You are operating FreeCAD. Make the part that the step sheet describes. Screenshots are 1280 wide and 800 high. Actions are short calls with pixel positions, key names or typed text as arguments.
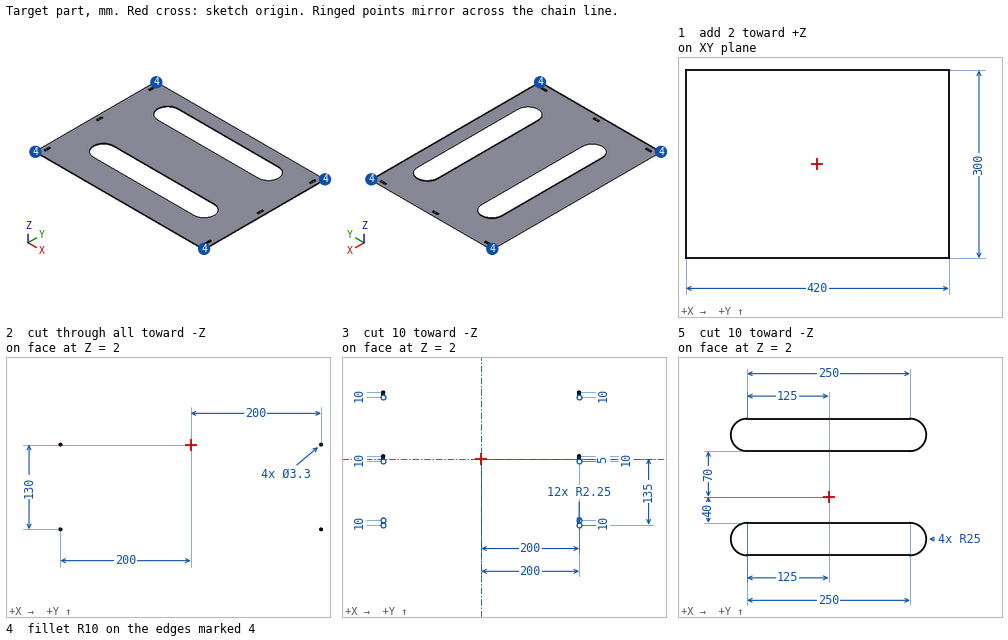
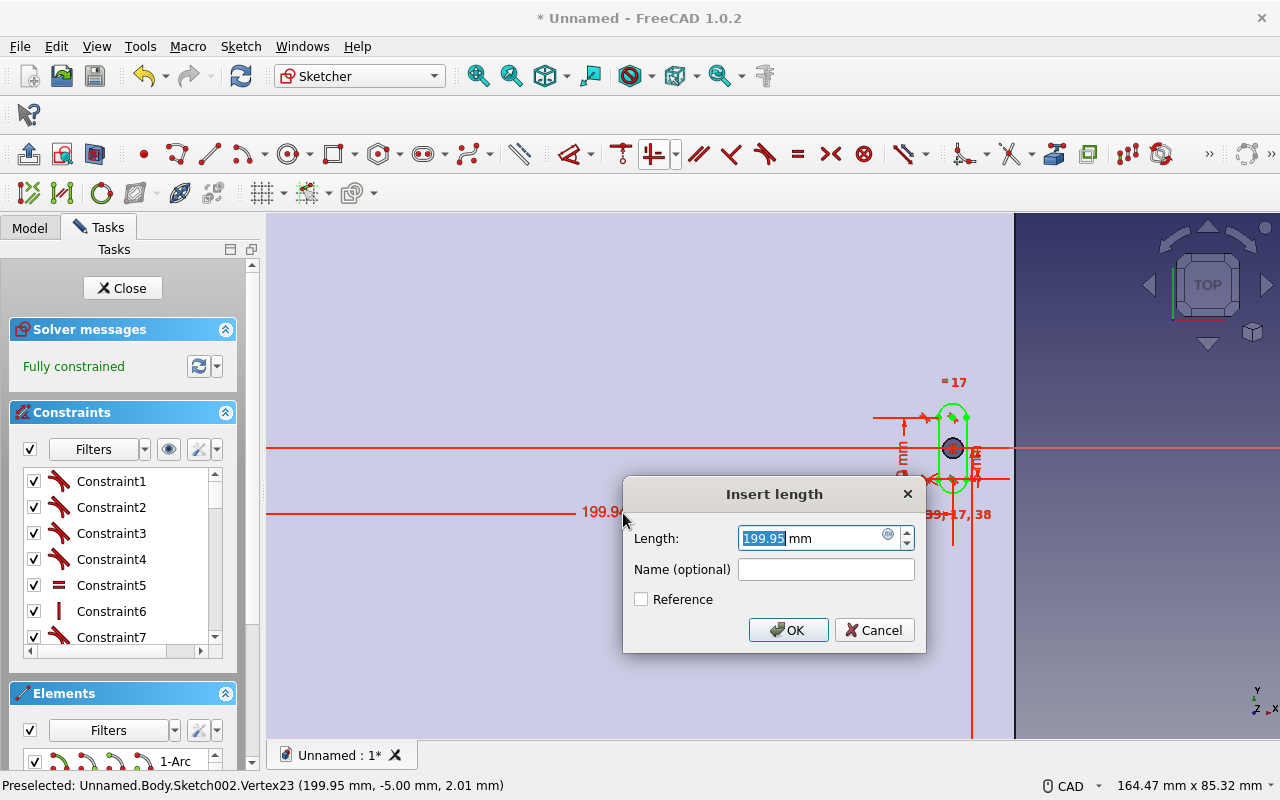
text(200)
key(Return)
key(Escape)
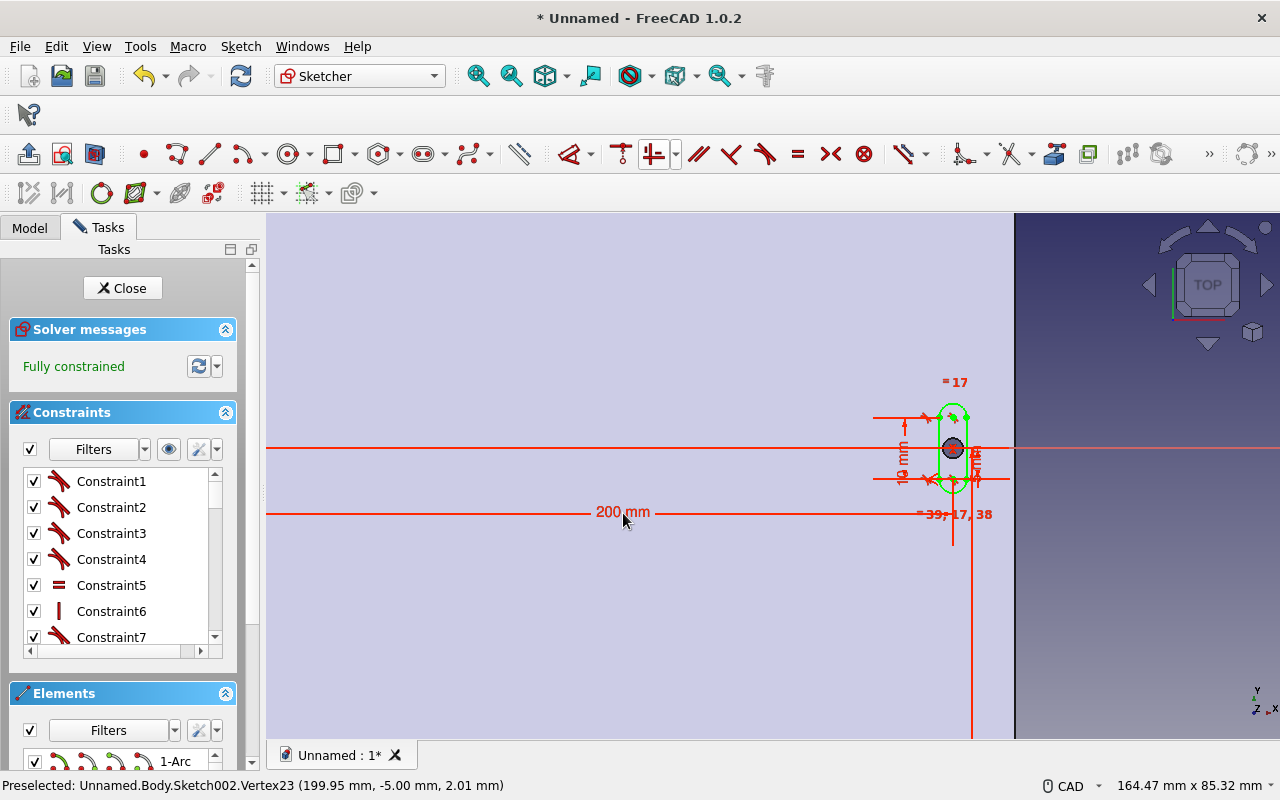
click(123, 288)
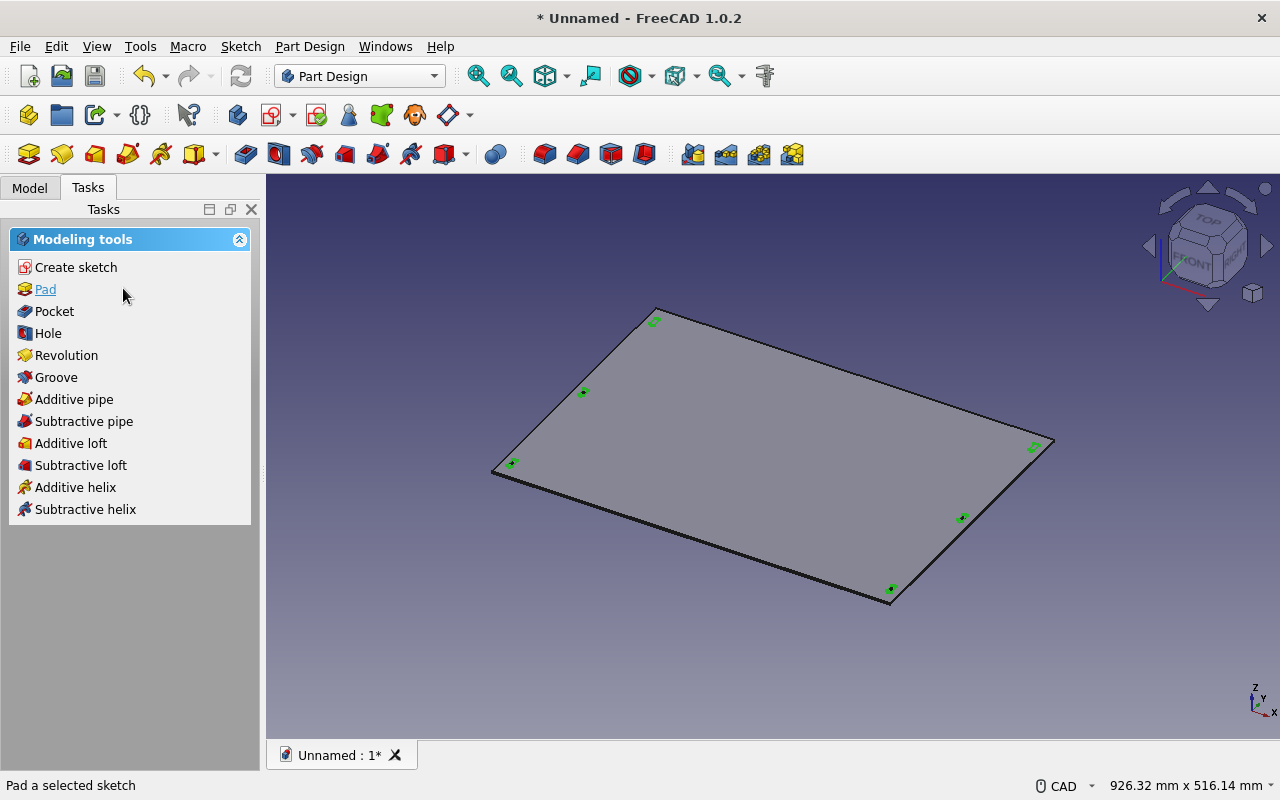
click(246, 154)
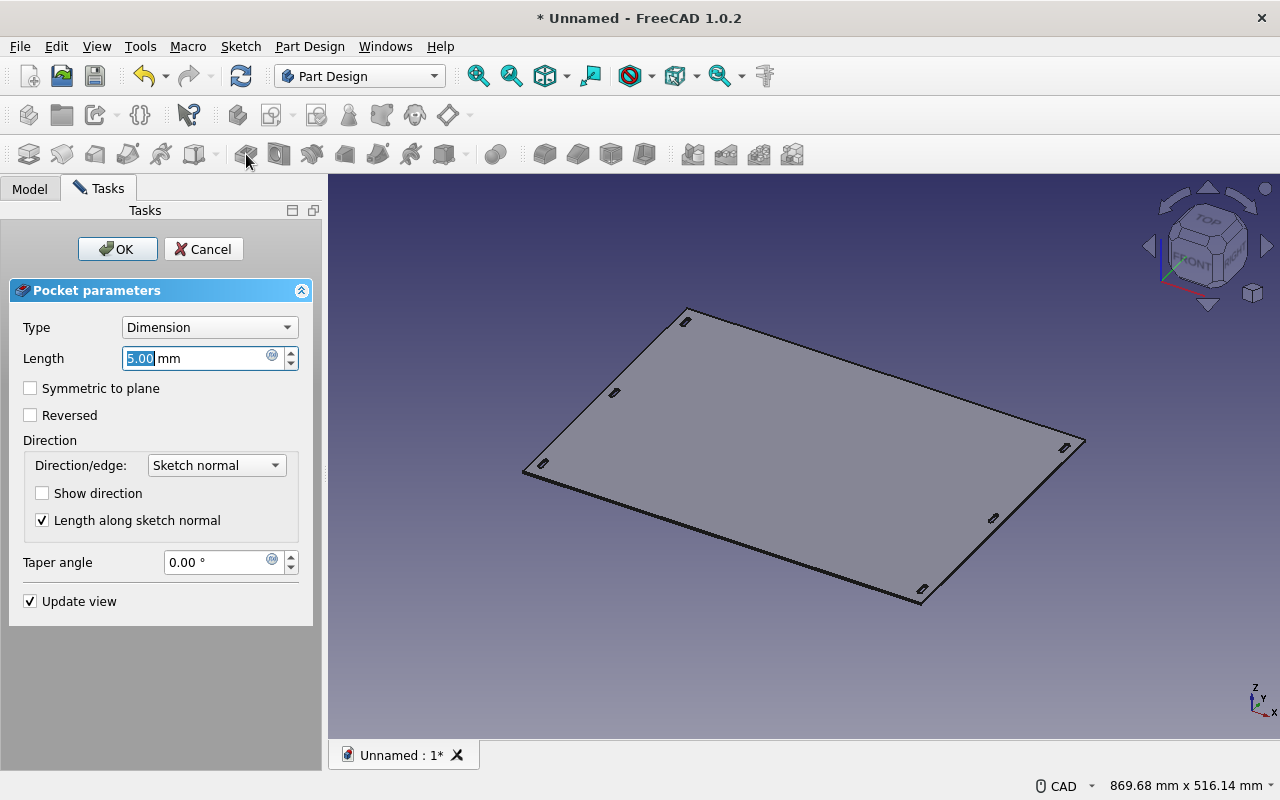
text(10)
key(Tab)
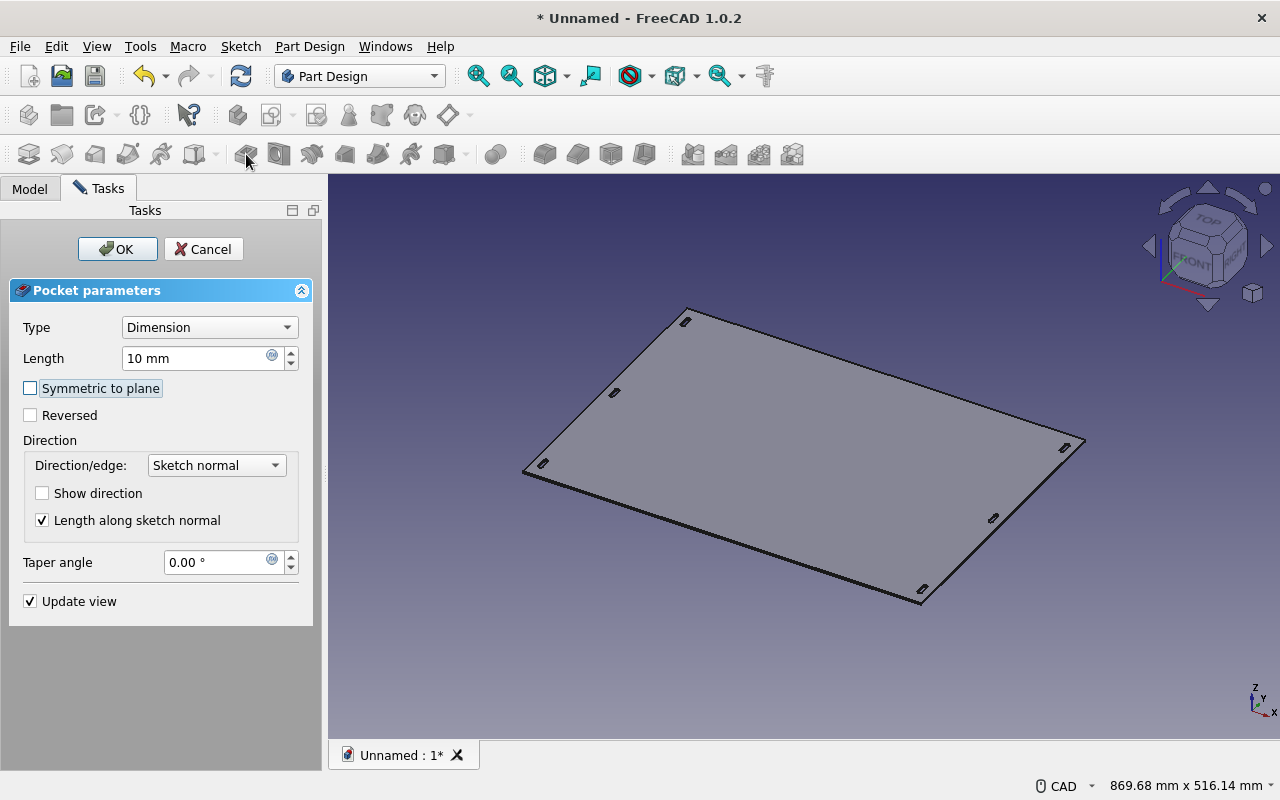
click(118, 249)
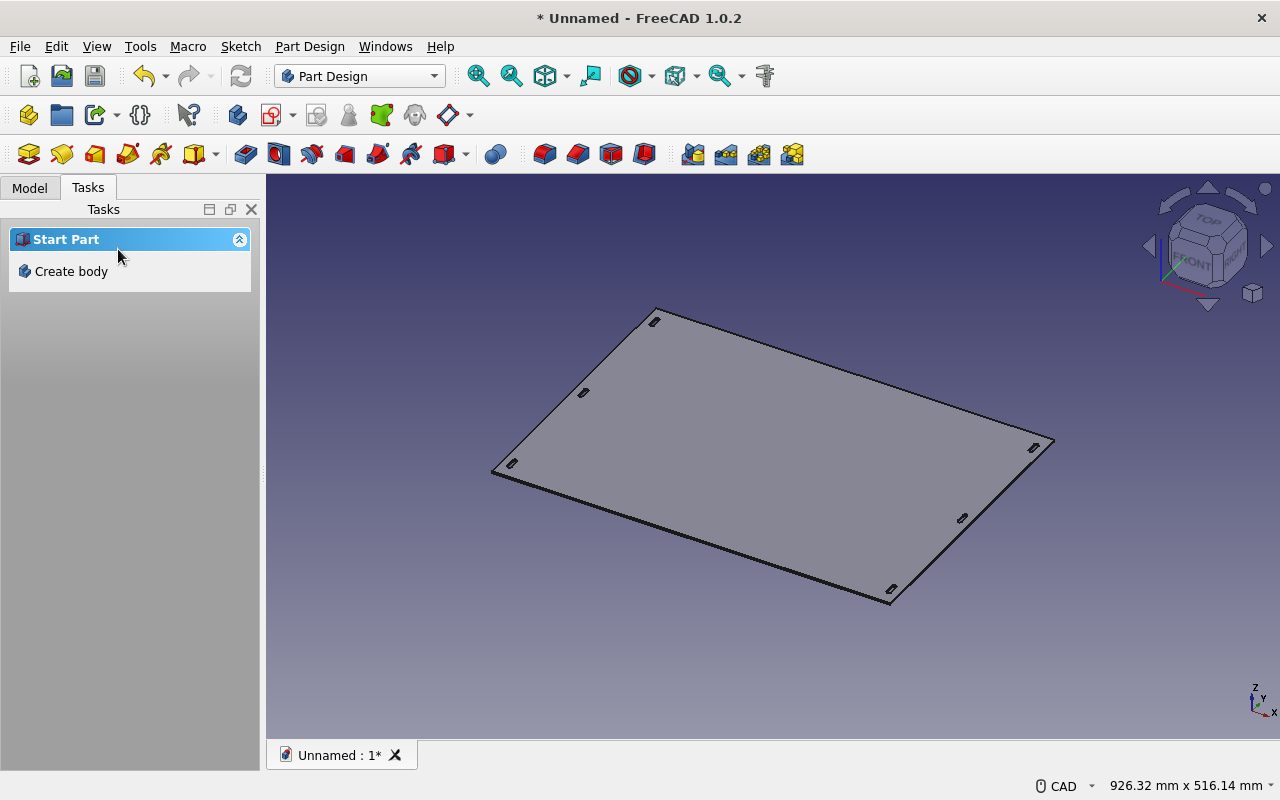
scroll(890, 603, up, 15)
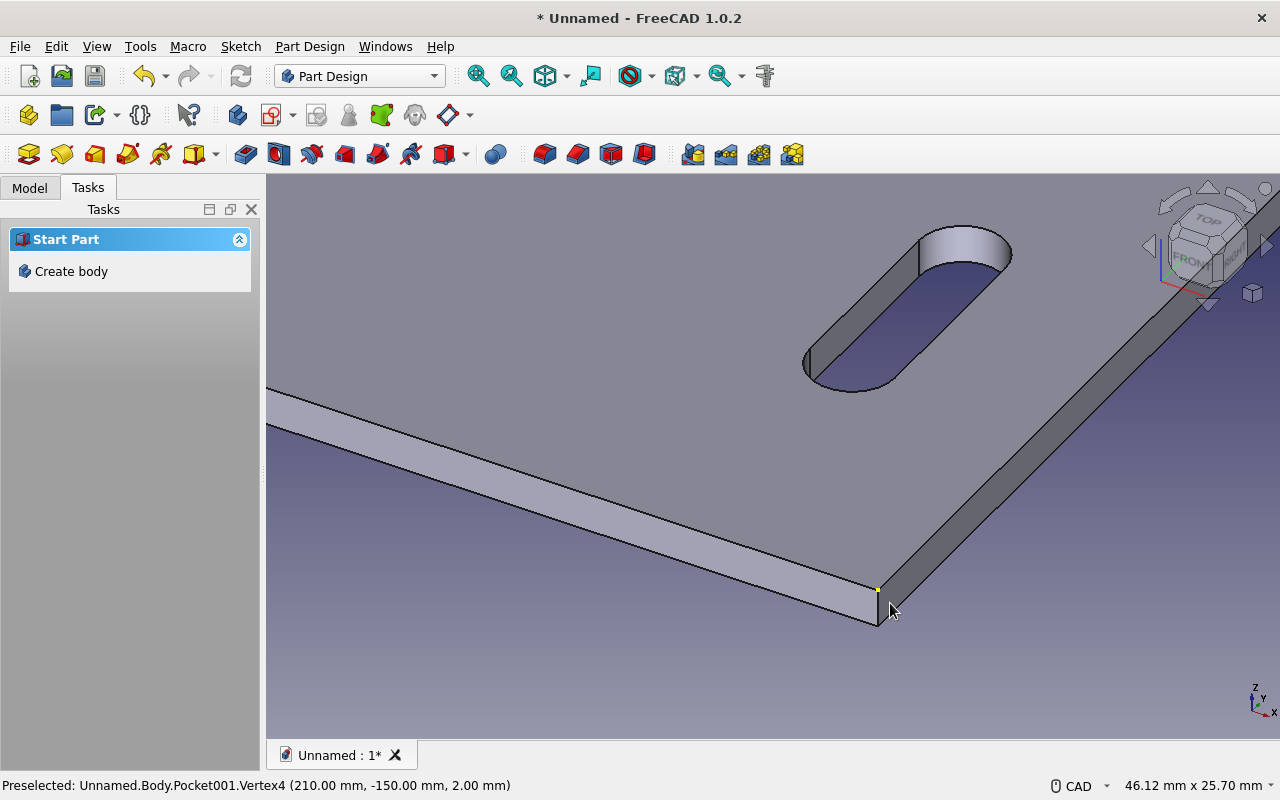
click(878, 607)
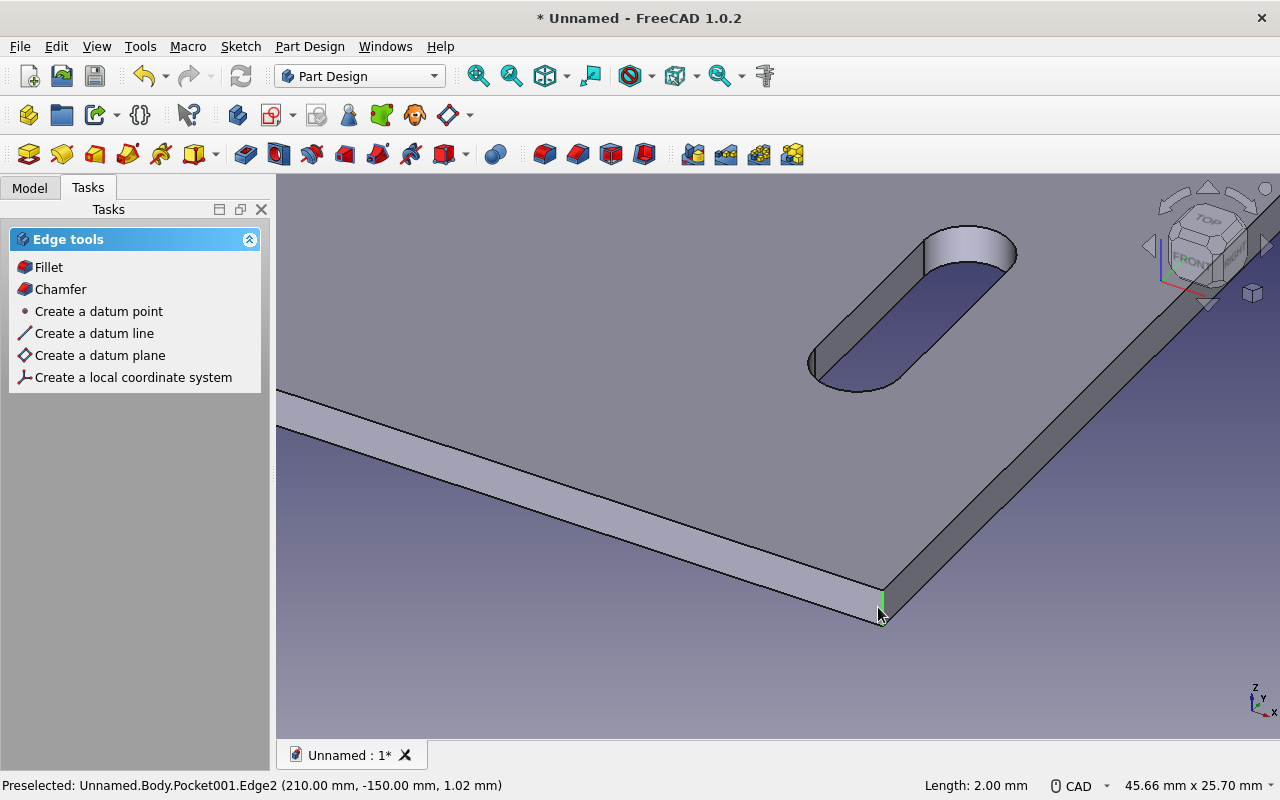
click(479, 76)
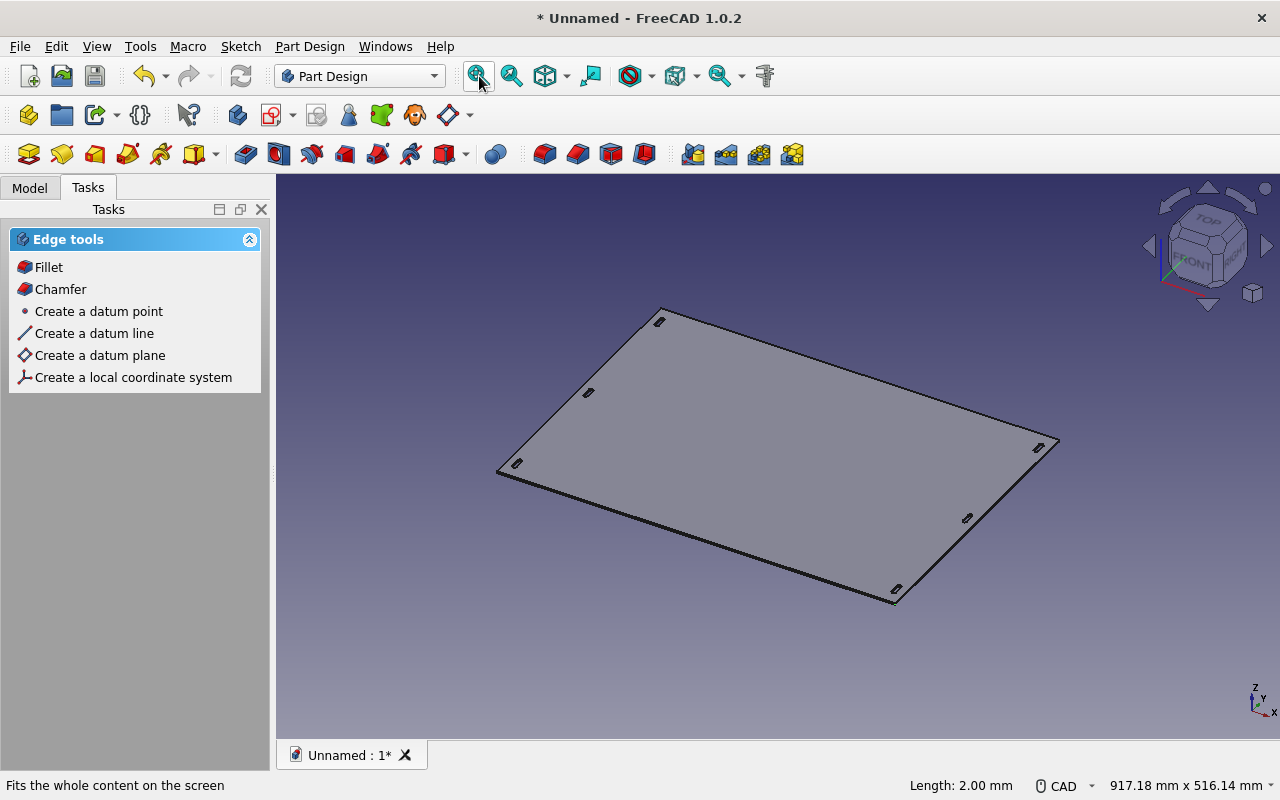
key(0)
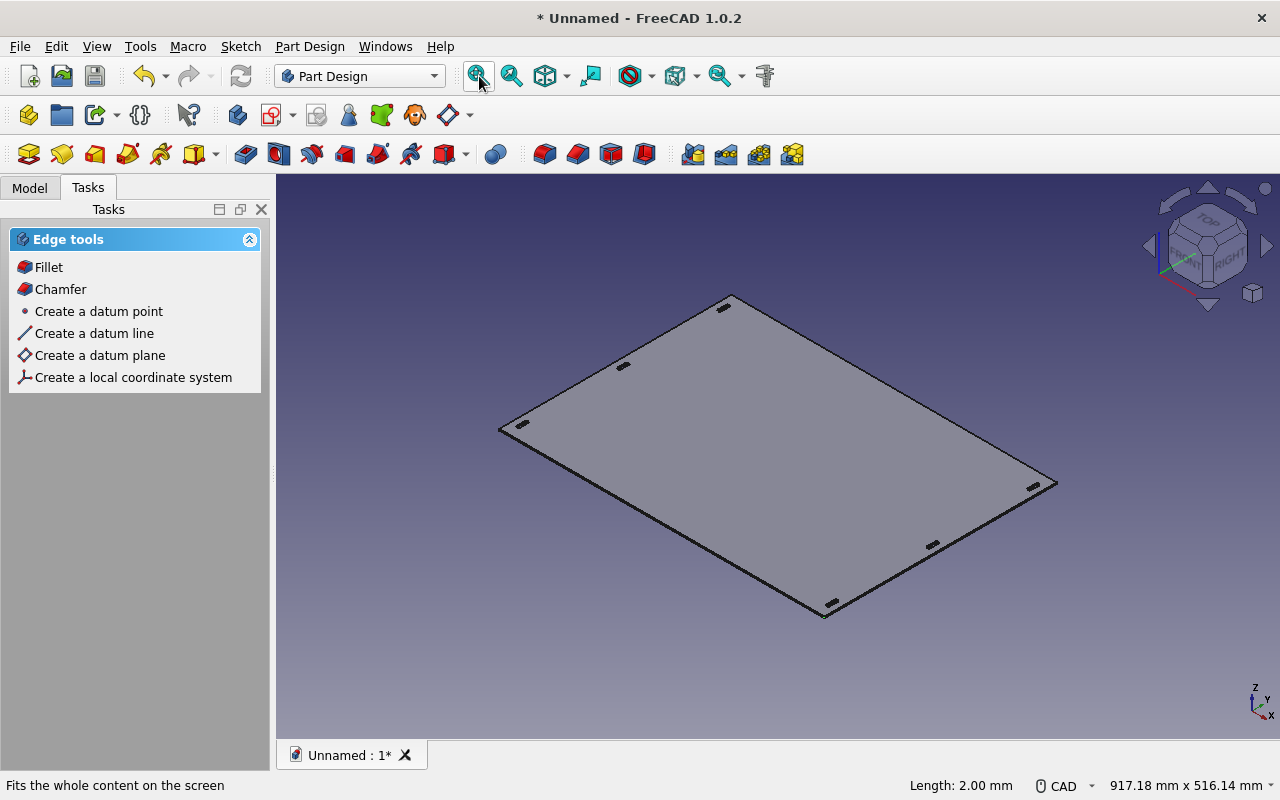
scroll(499, 429, up, 15)